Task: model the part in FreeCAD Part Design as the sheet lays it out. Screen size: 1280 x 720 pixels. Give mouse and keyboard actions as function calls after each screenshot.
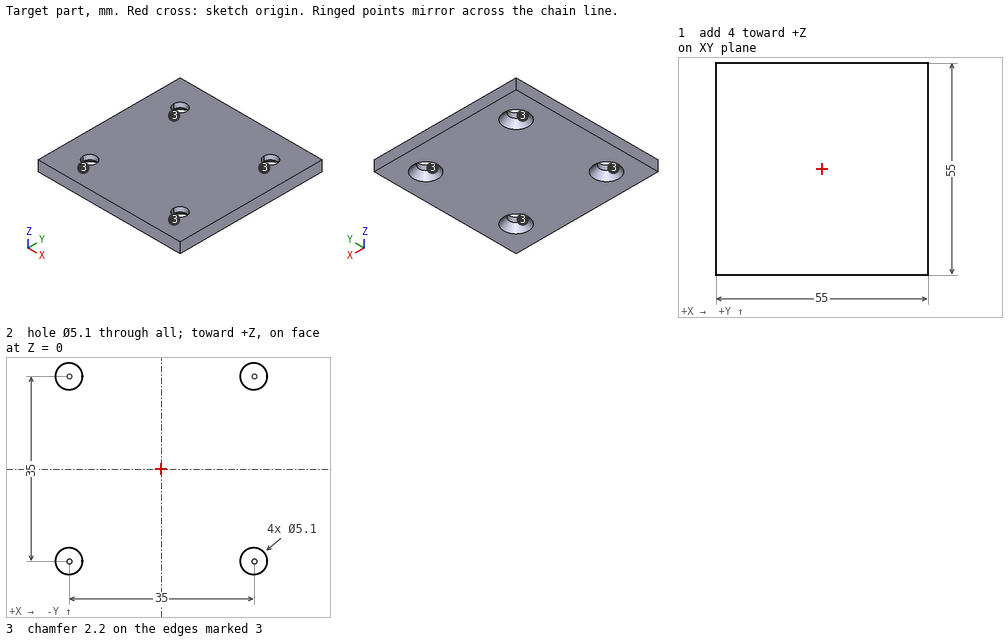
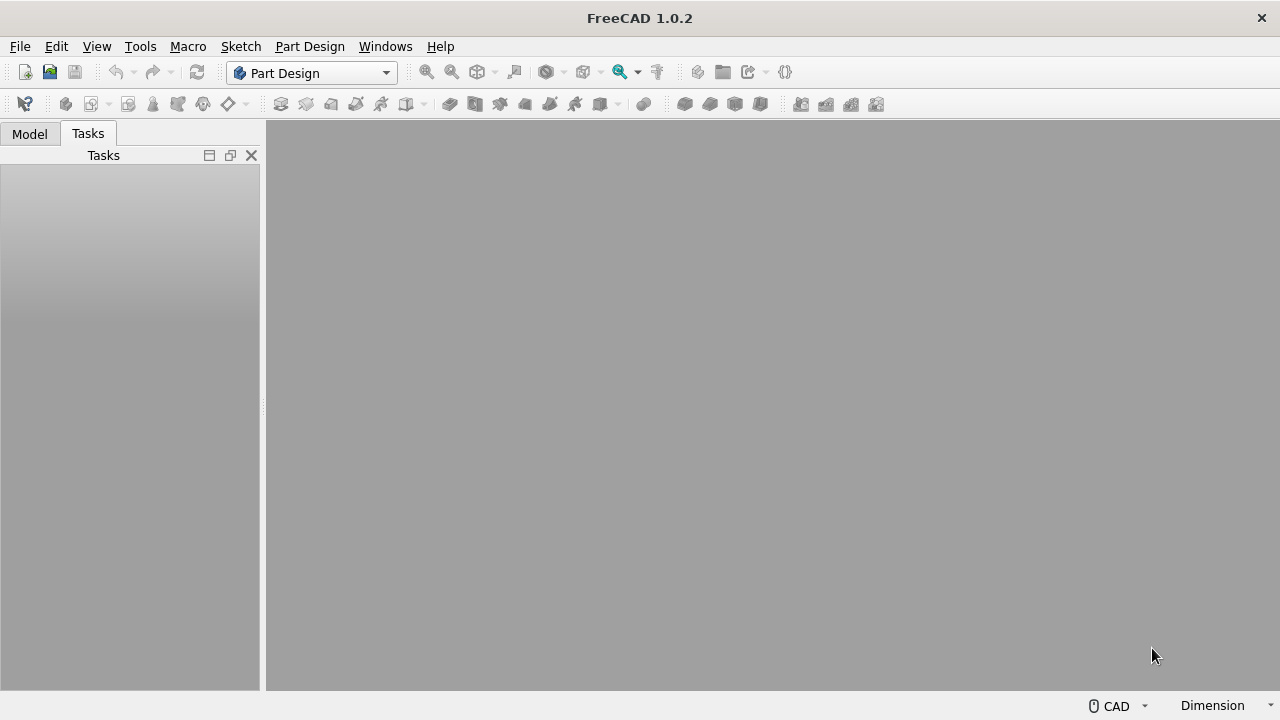
click(25, 72)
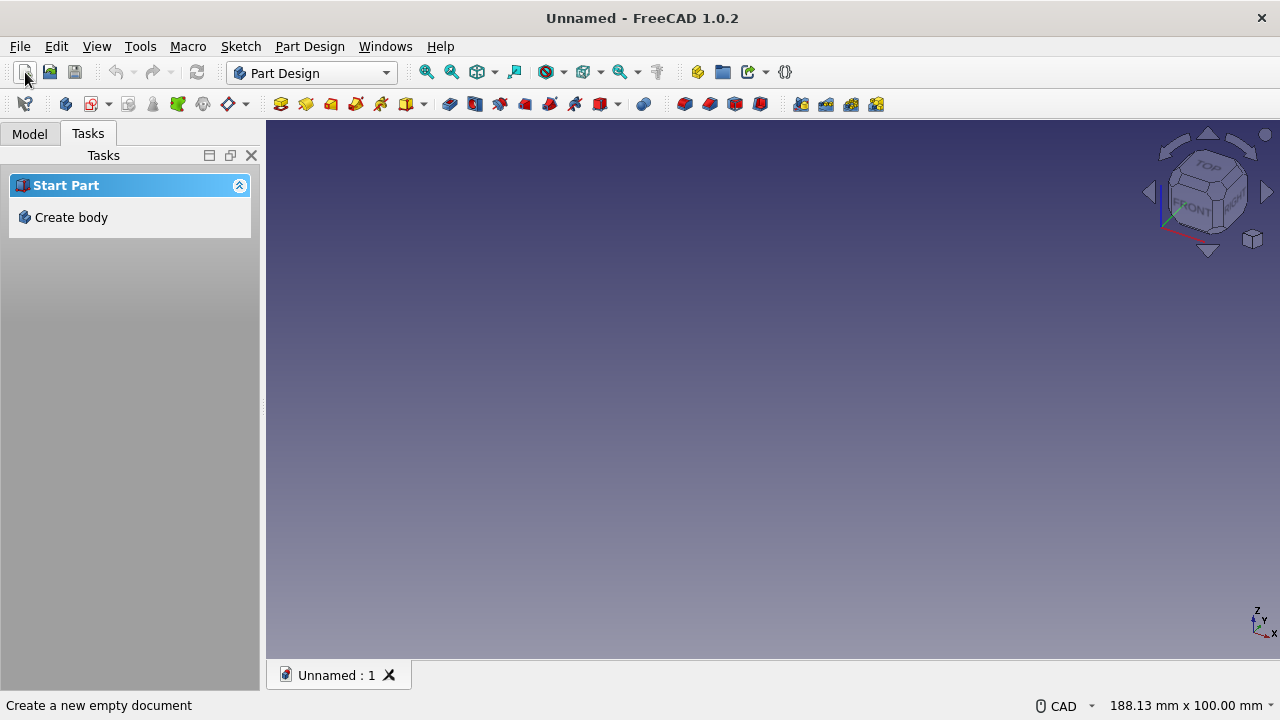
click(90, 104)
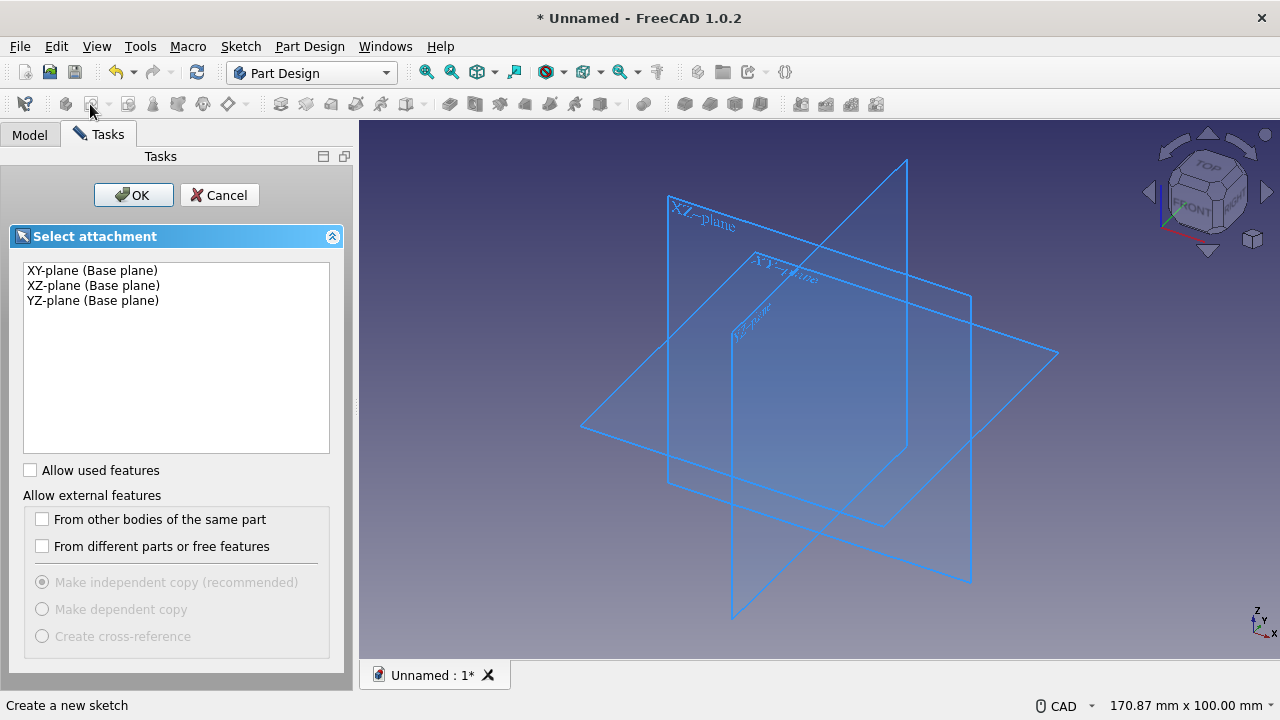
click(84, 270)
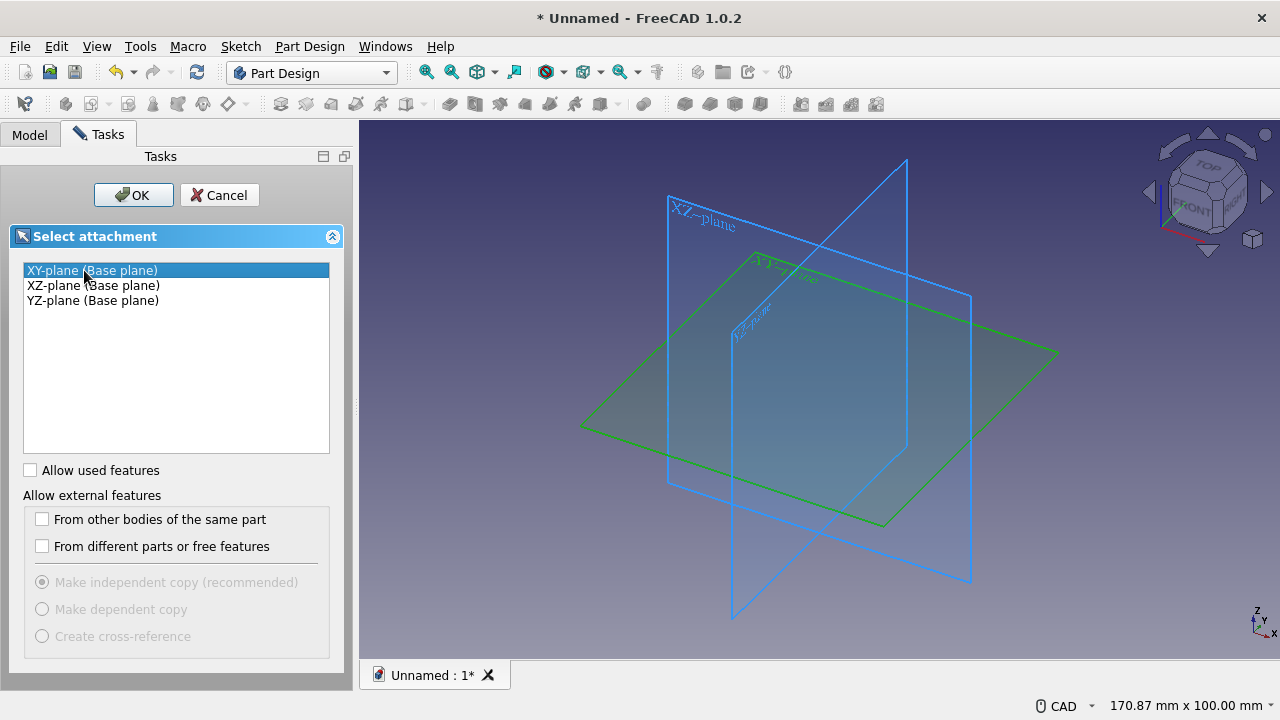
click(134, 195)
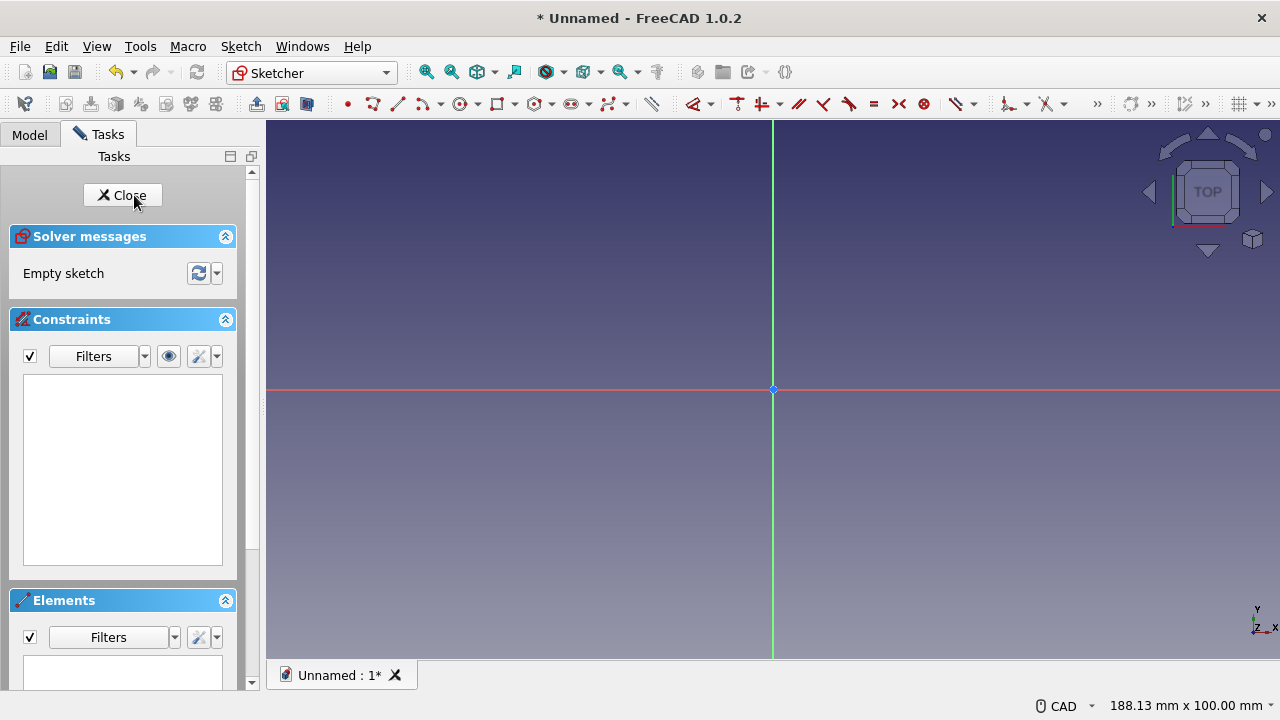
click(514, 104)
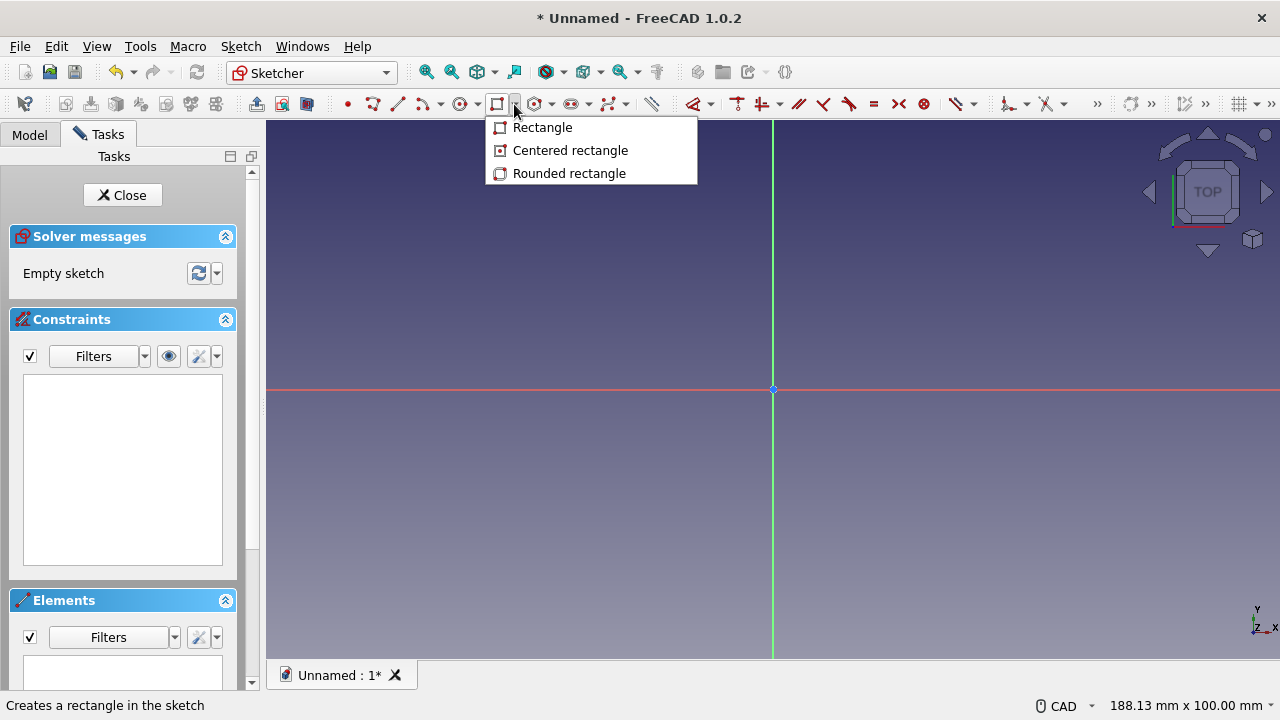
click(592, 150)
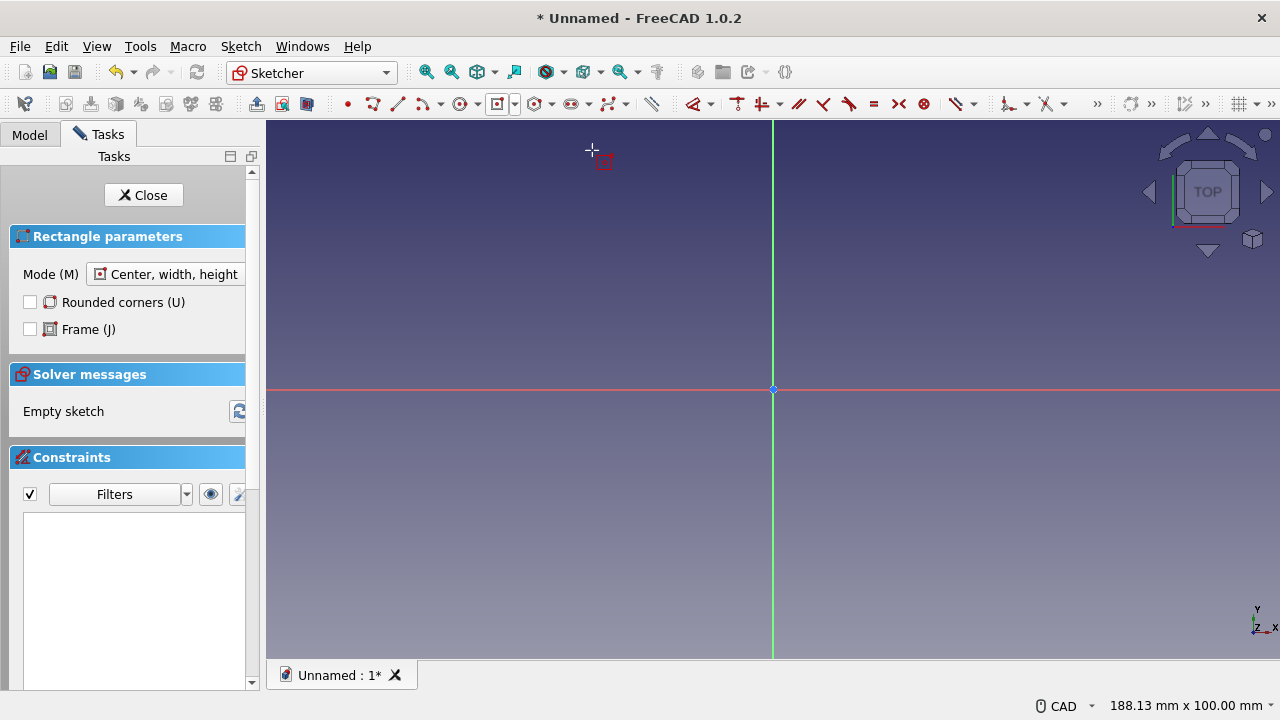
click(773, 390)
move(921, 241)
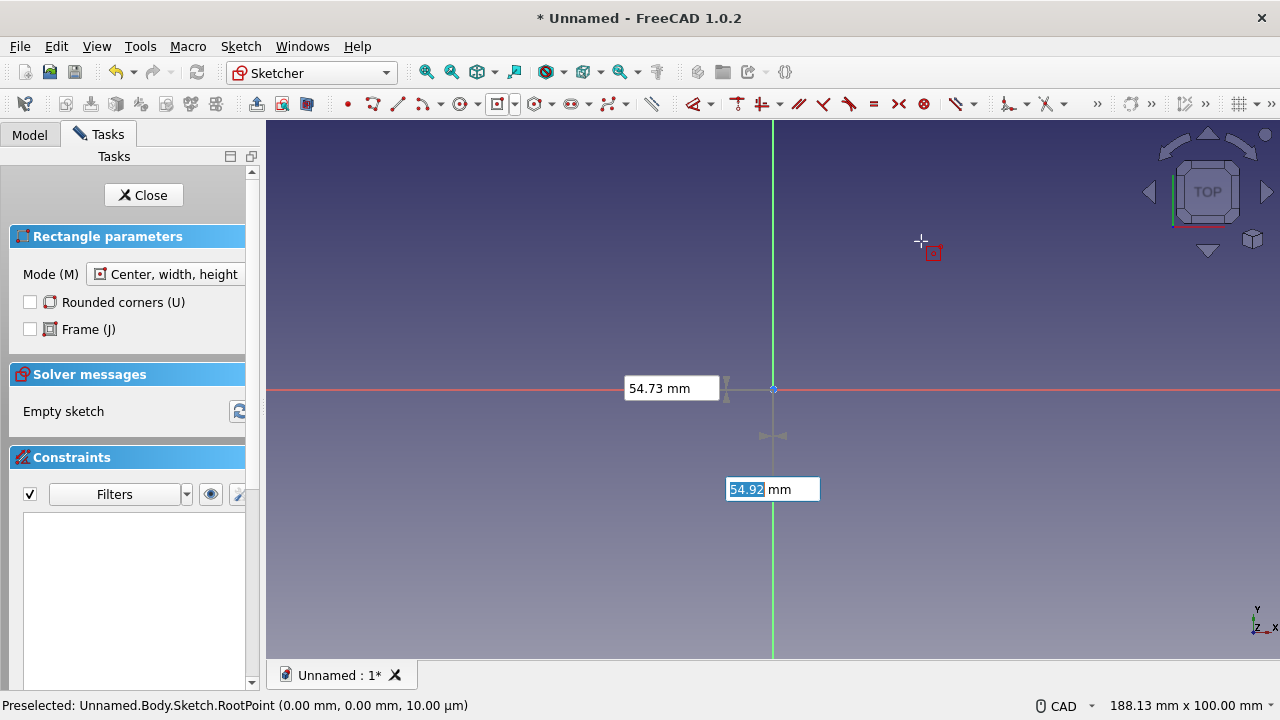
text(55)
key(Tab)
text(55)
key(Return)
key(Escape)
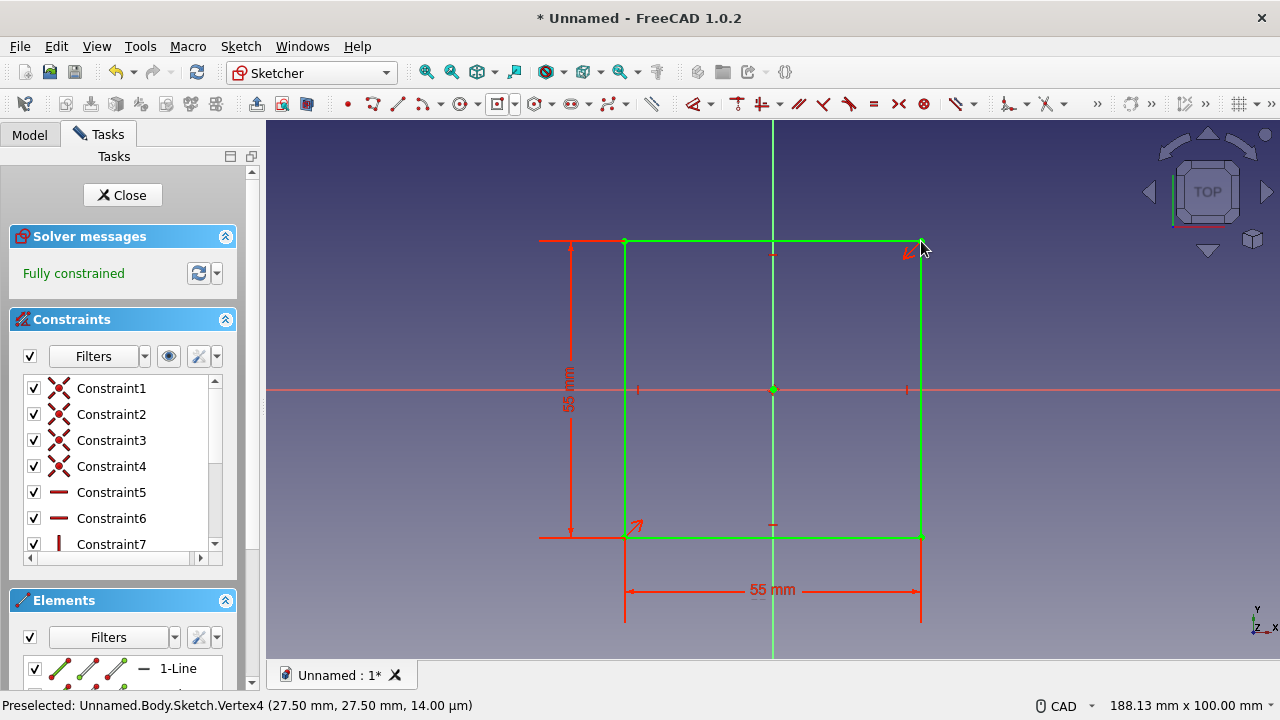
click(123, 195)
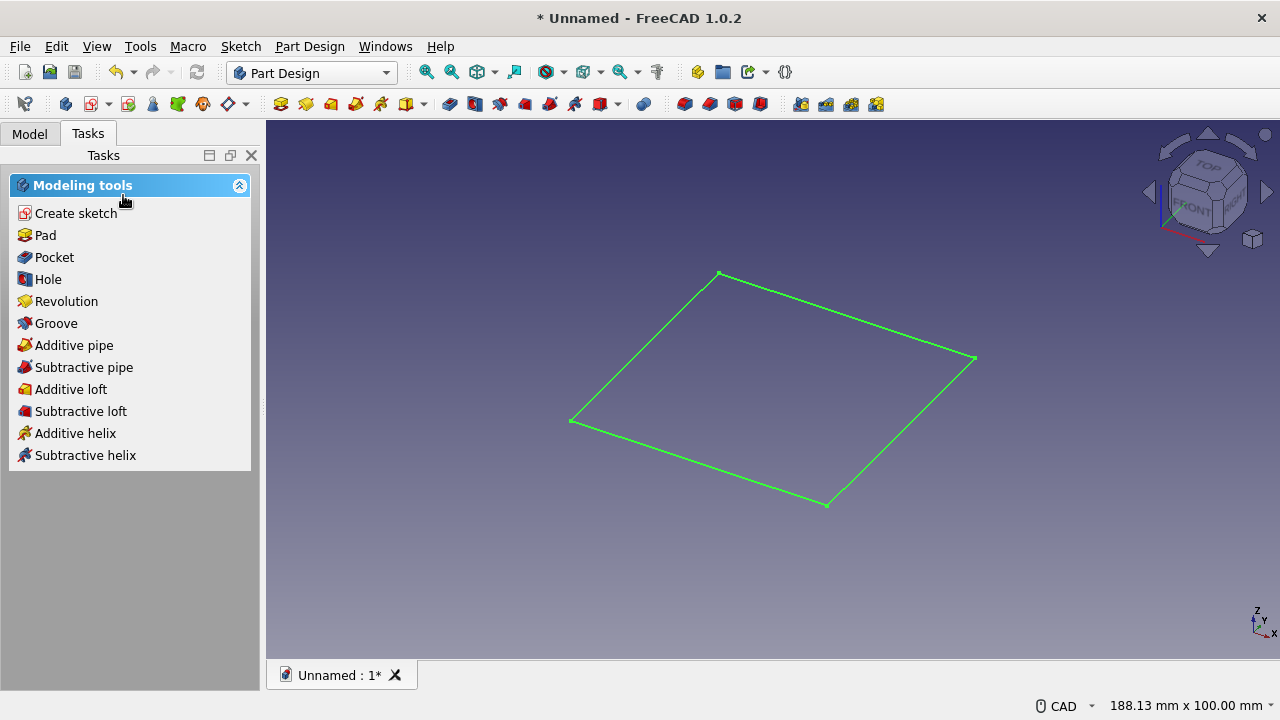
click(281, 104)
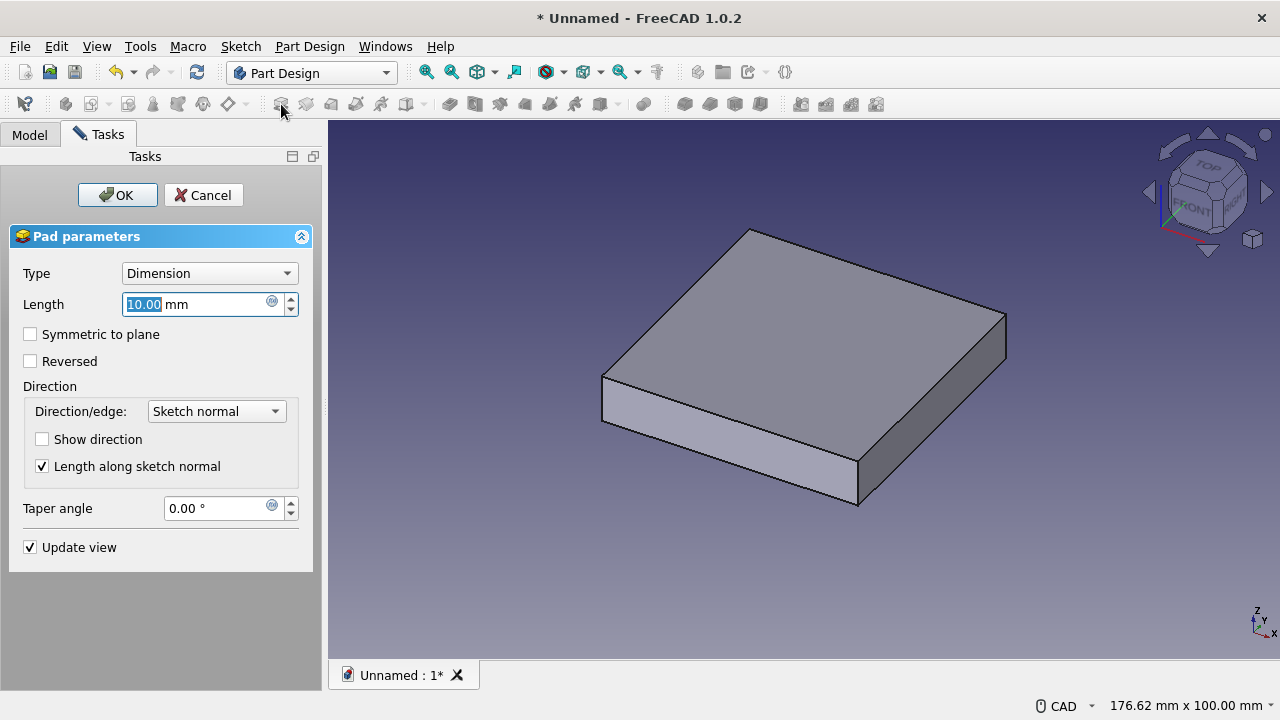
text(4)
key(Tab)